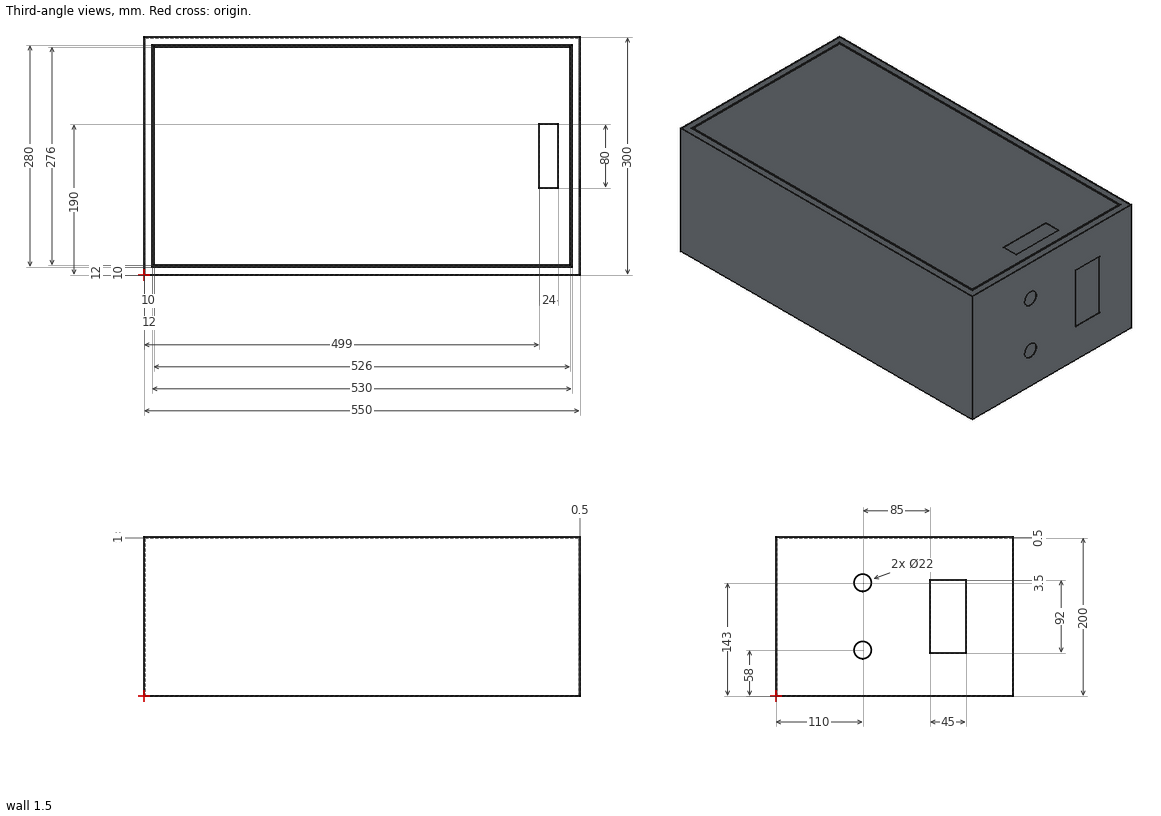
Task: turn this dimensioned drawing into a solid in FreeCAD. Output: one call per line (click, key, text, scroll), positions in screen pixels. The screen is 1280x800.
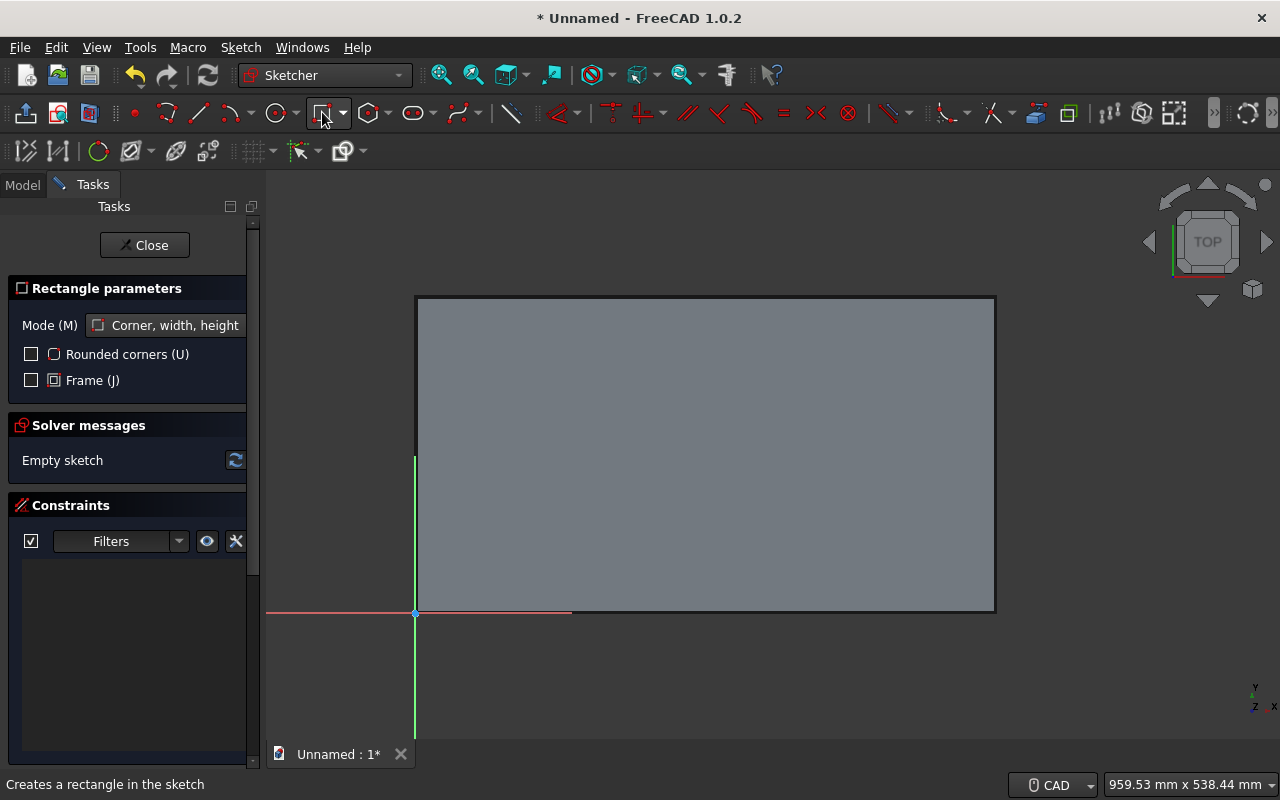
click(415, 613)
move(996, 296)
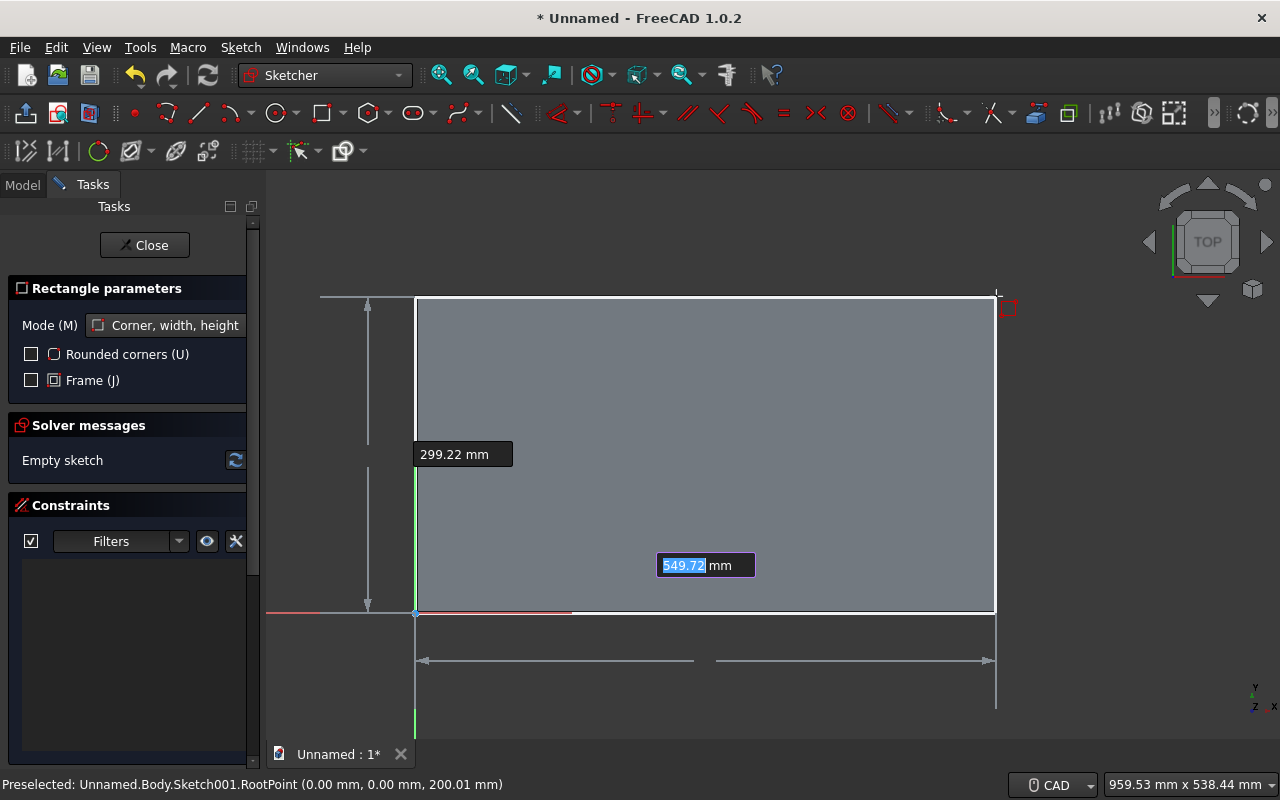
text(550)
key(Tab)
text(300)
key(Return)
key(Escape)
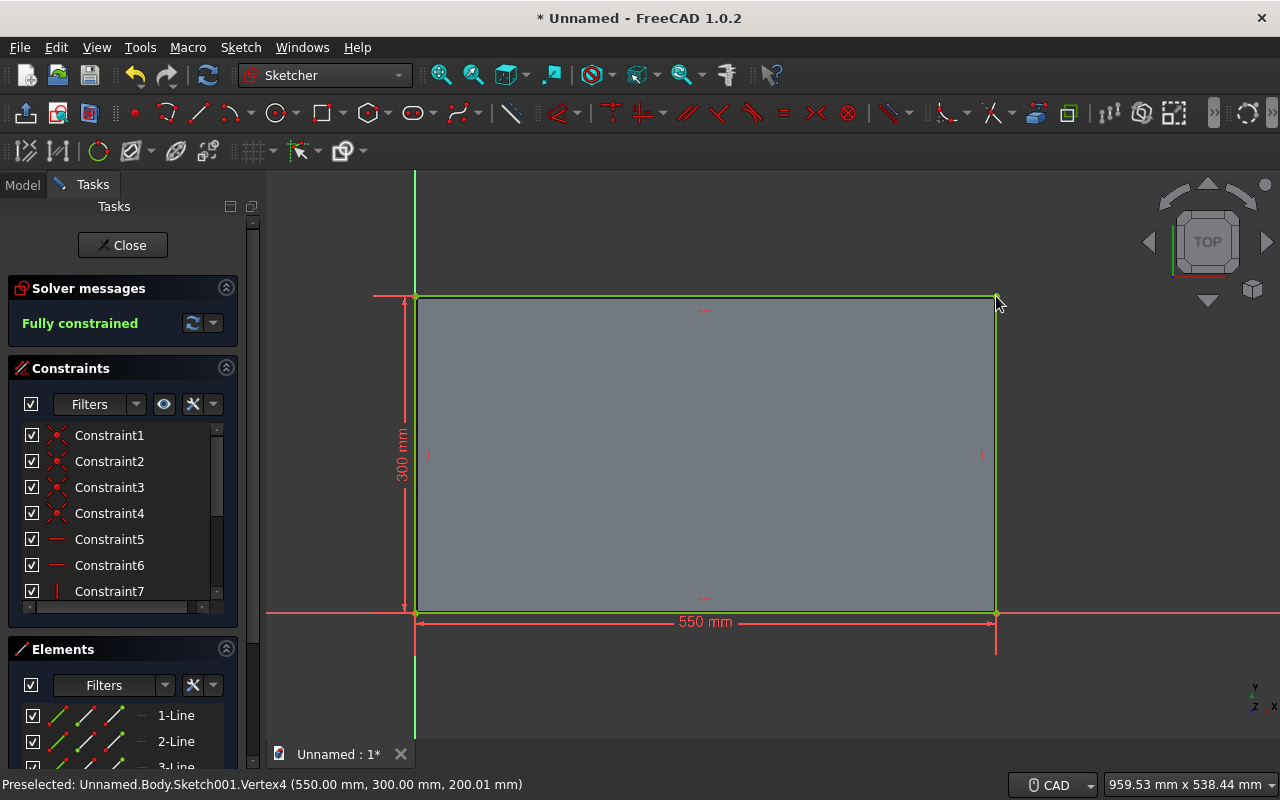
click(123, 245)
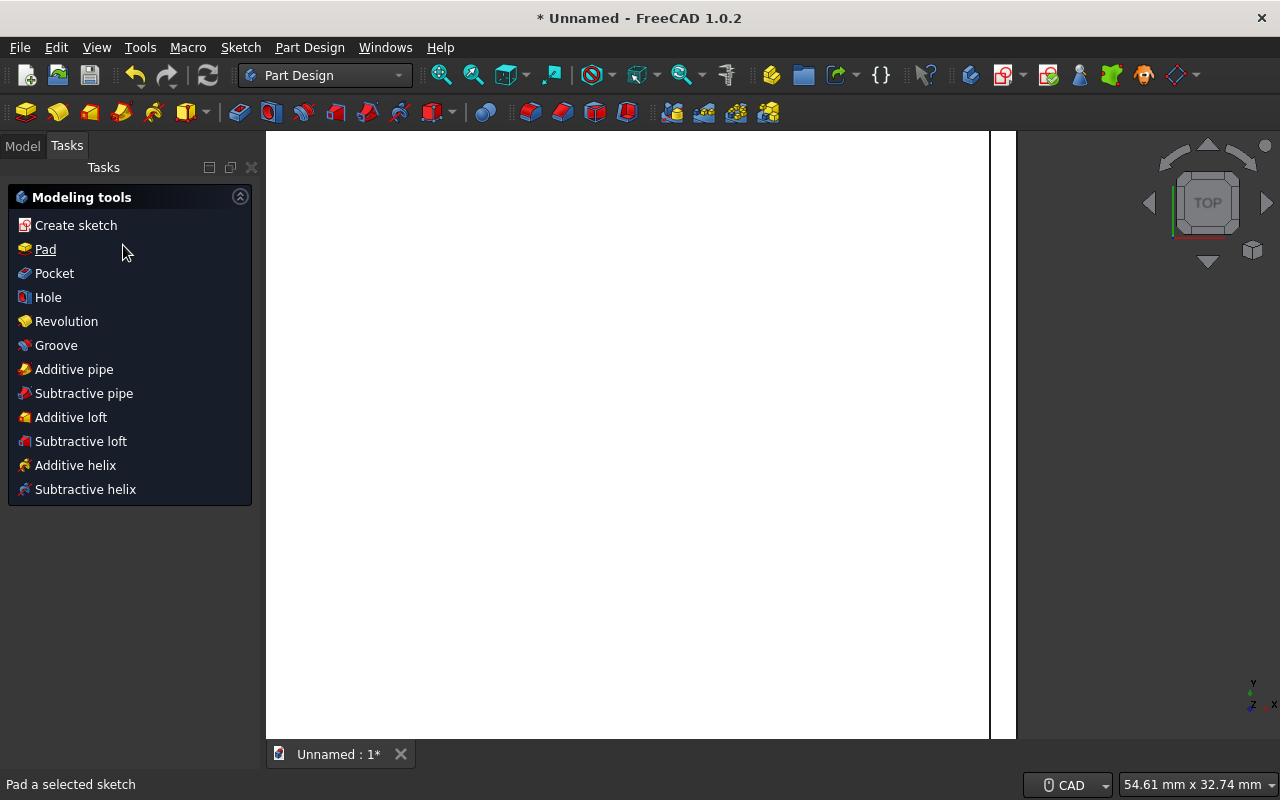
click(26, 112)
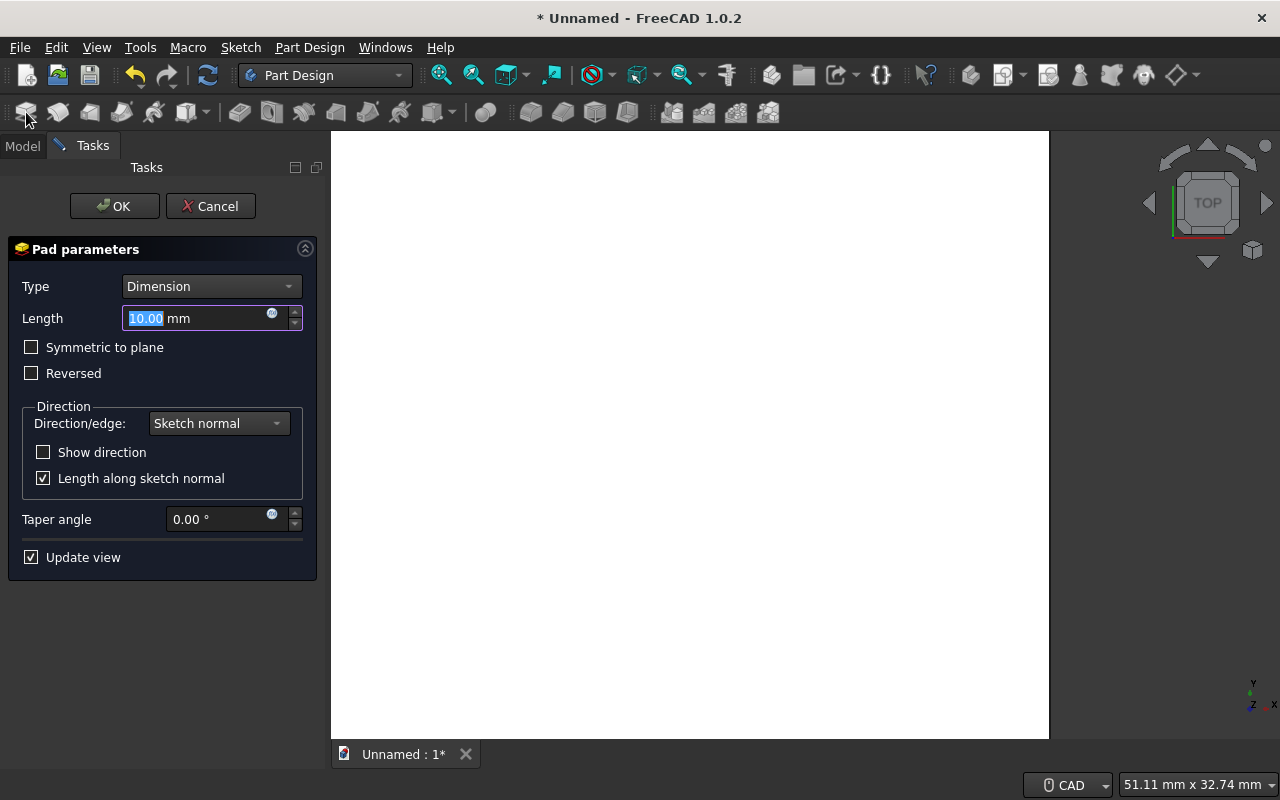
text(1)
key(Tab)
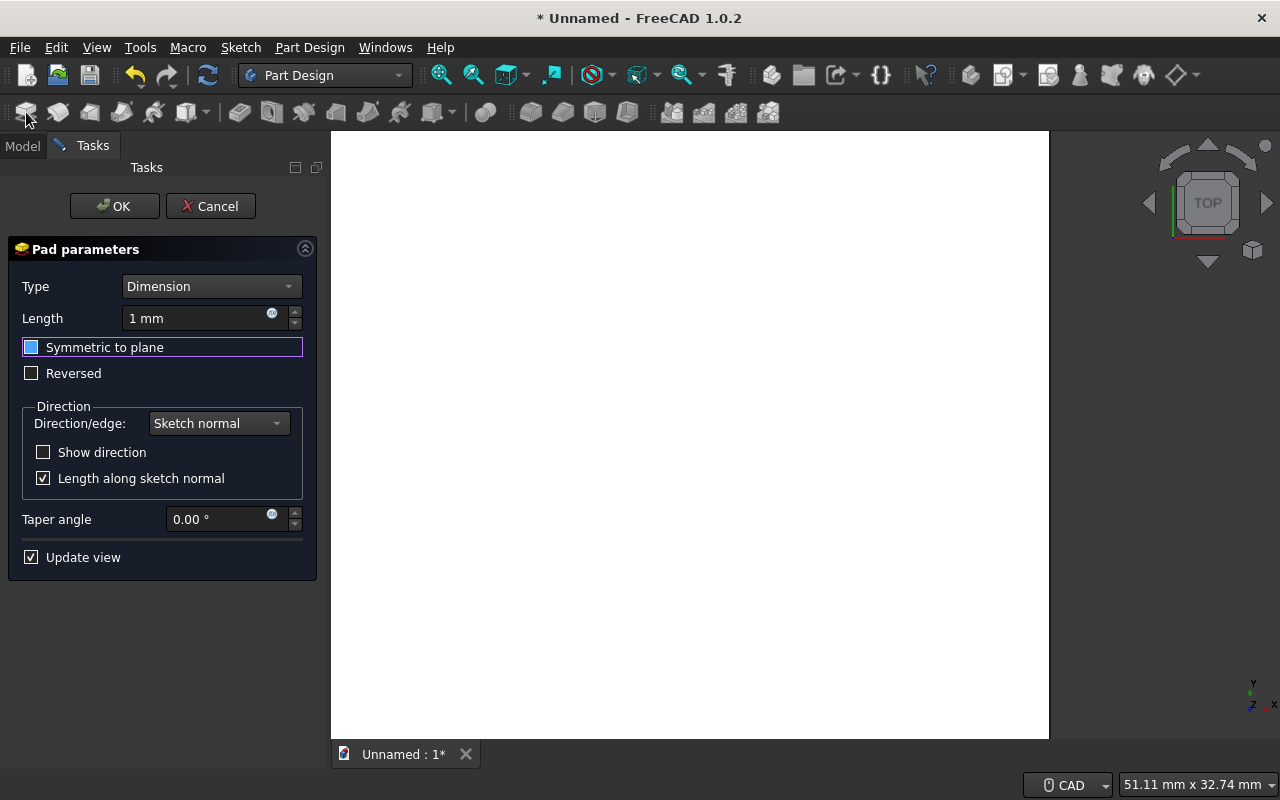
click(115, 206)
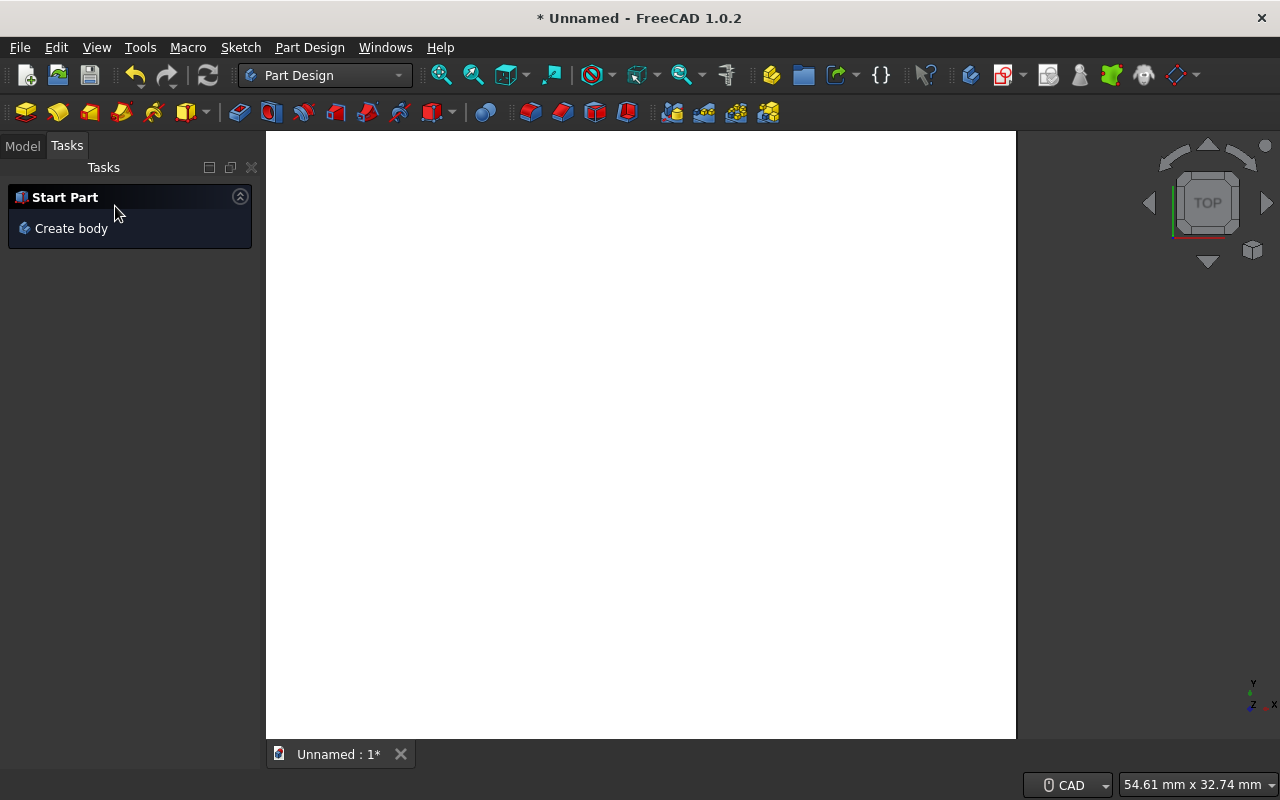
click(442, 76)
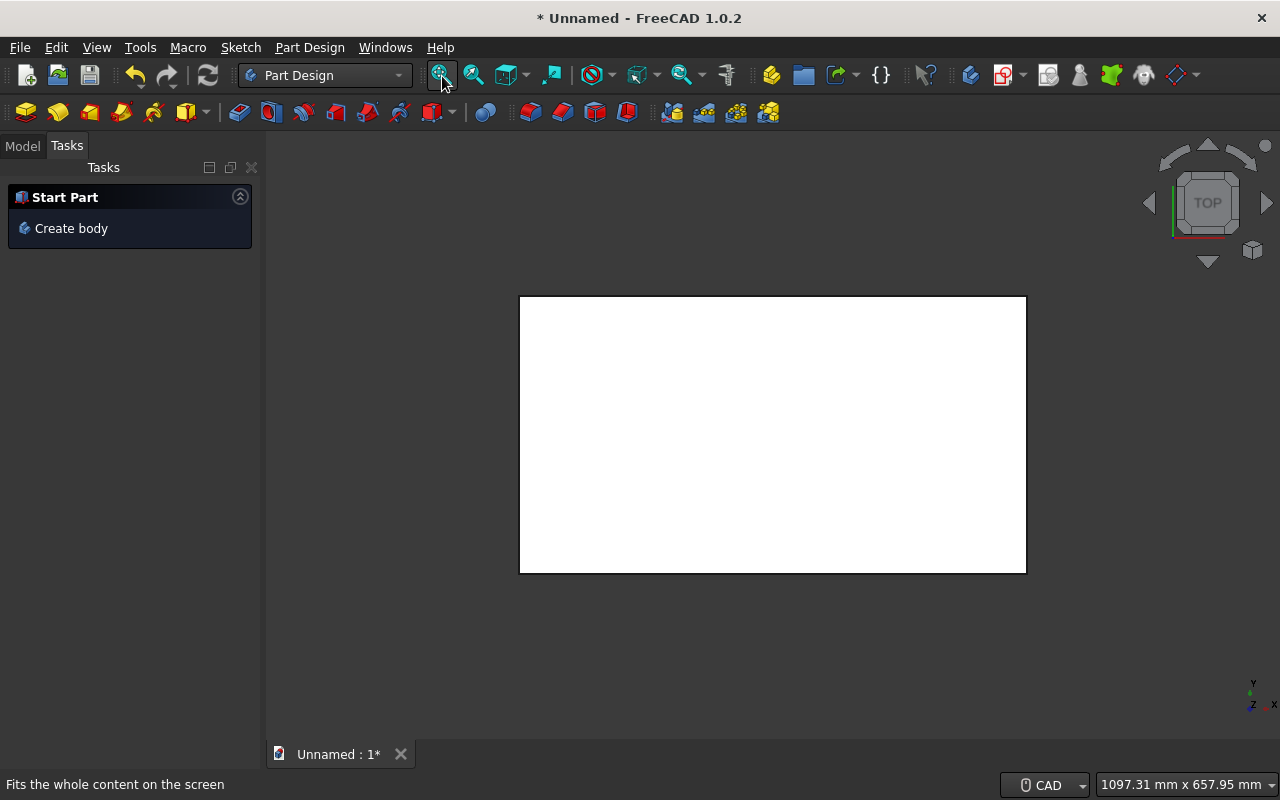
click(846, 434)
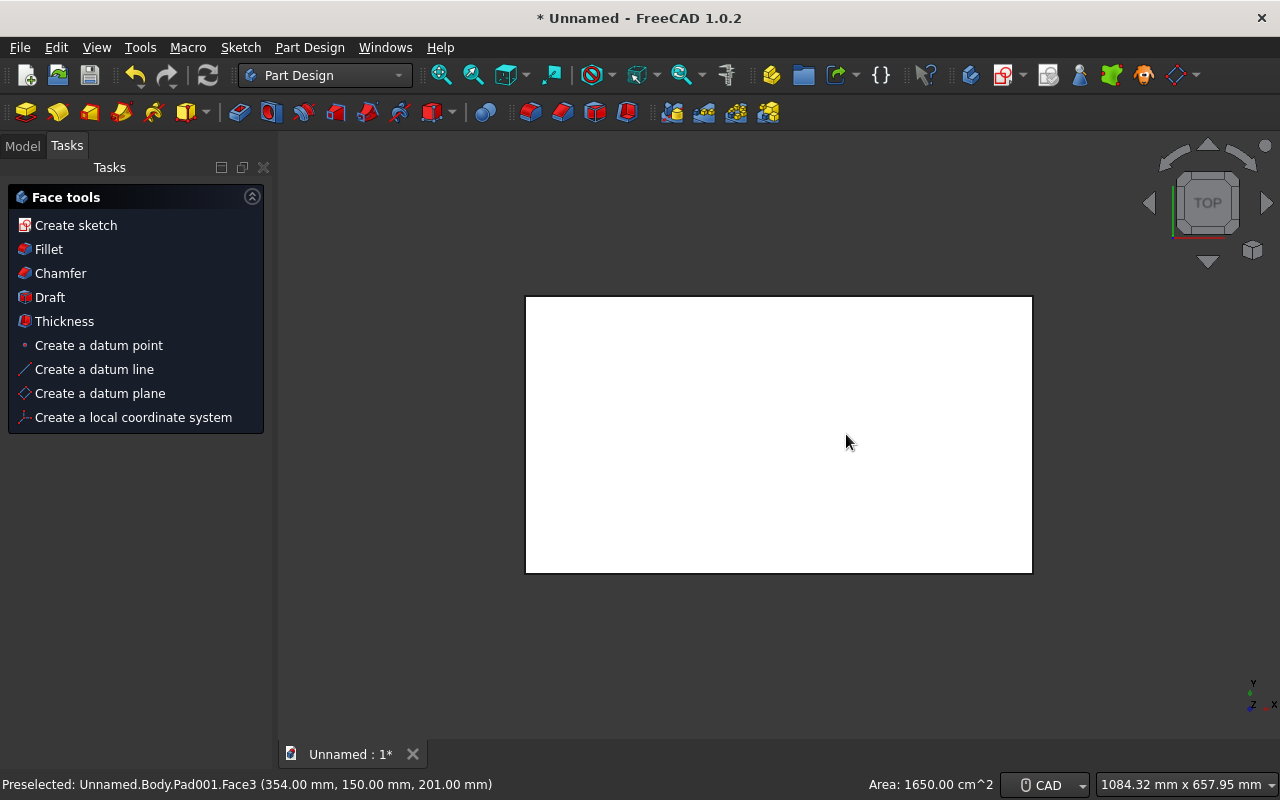
click(1004, 76)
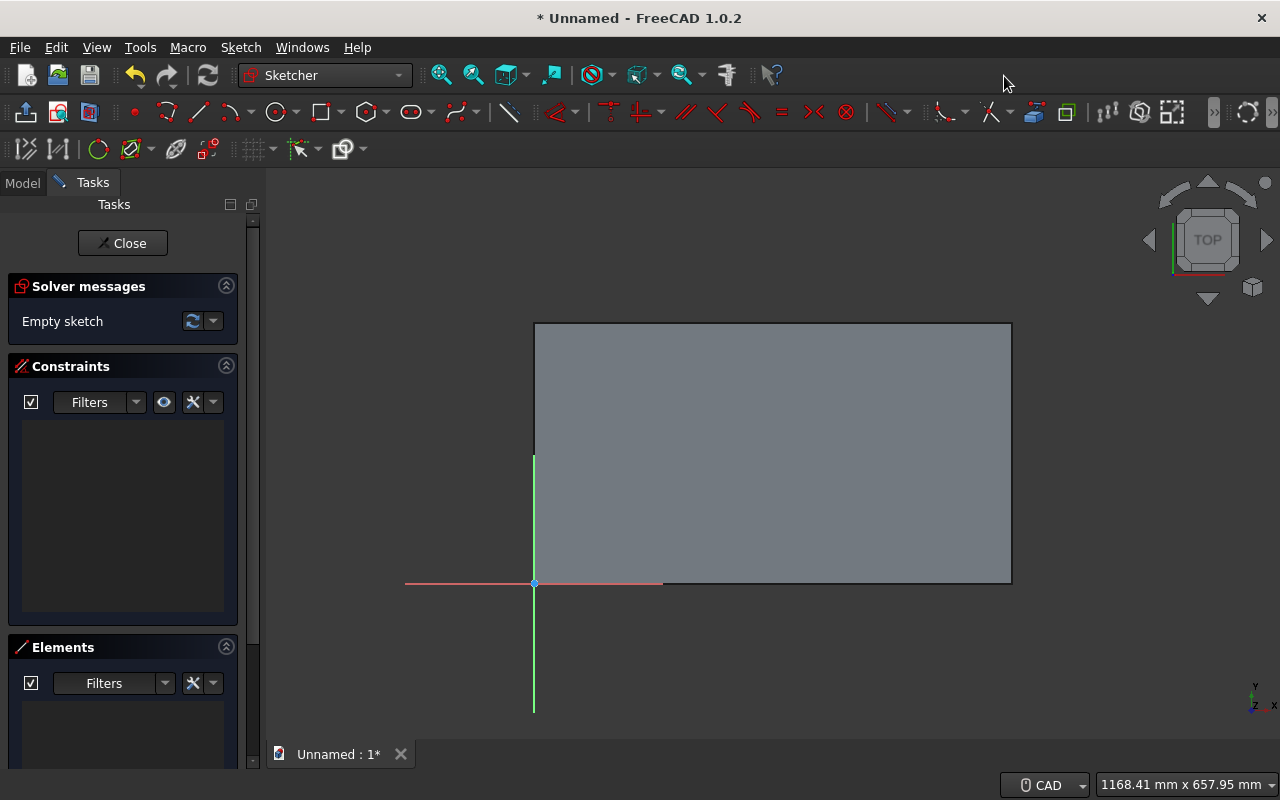
click(322, 112)